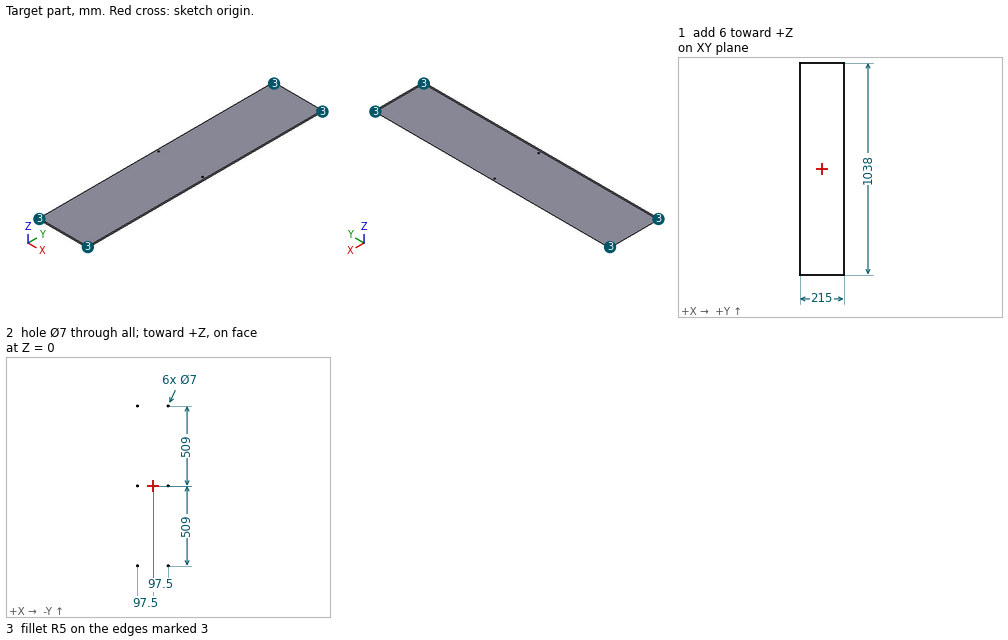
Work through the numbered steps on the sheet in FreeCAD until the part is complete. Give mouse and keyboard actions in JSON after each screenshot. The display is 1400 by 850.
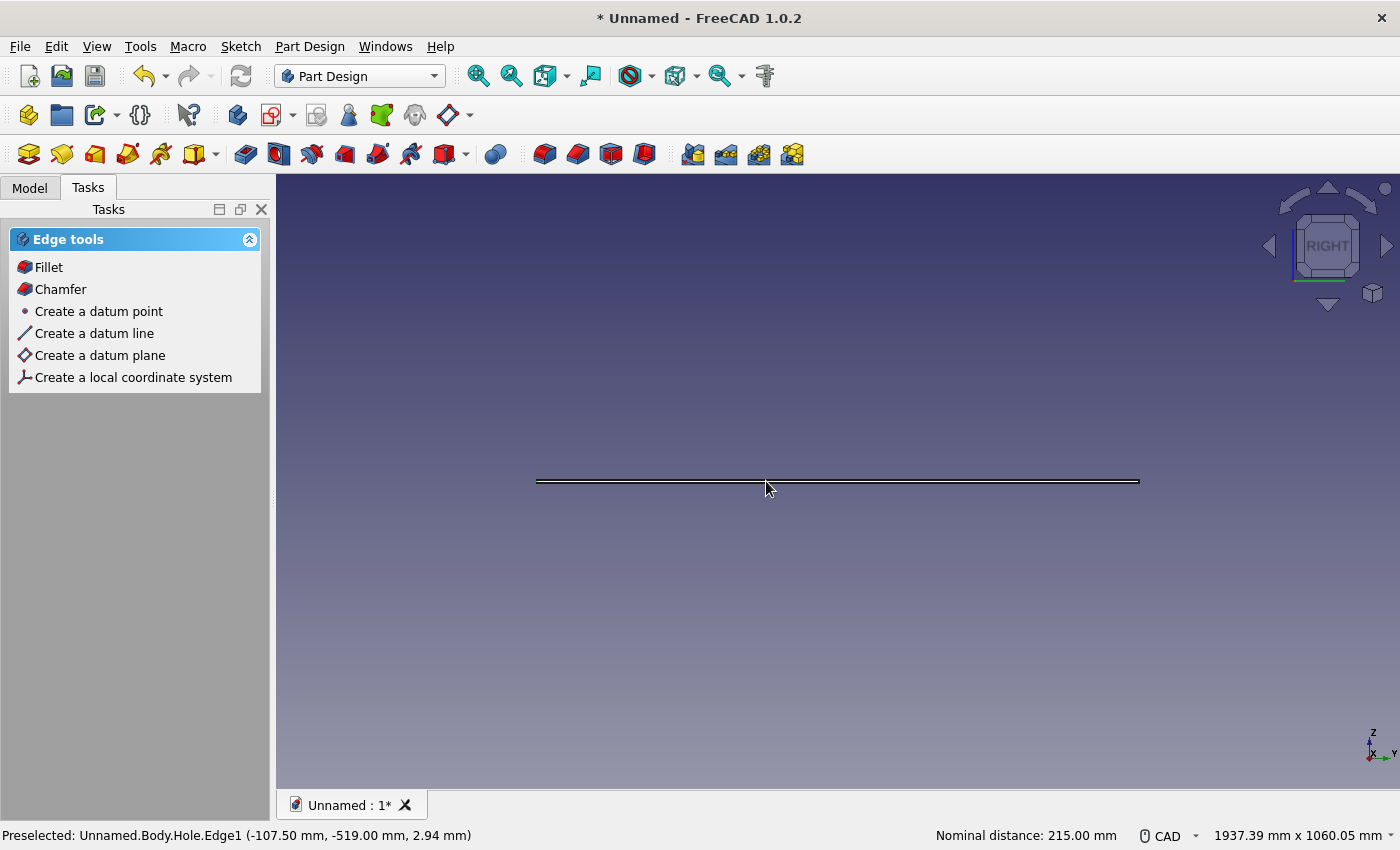
{"action": "scroll", "coordinate": [1139, 480], "scroll_direction": "up", "scroll_amount": 13}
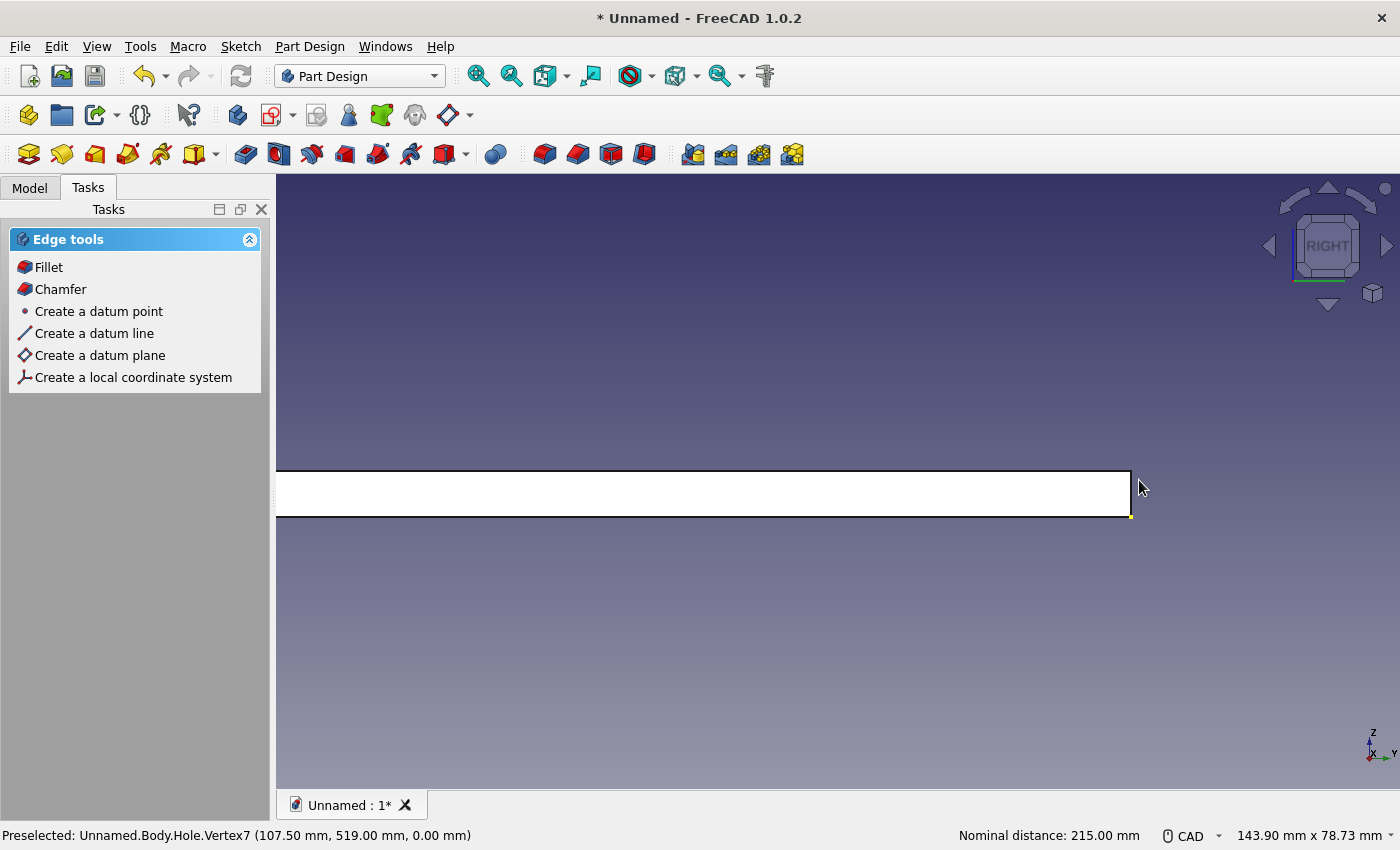
{"action": "left_click", "coordinate": [1131, 493], "text": "ctrl"}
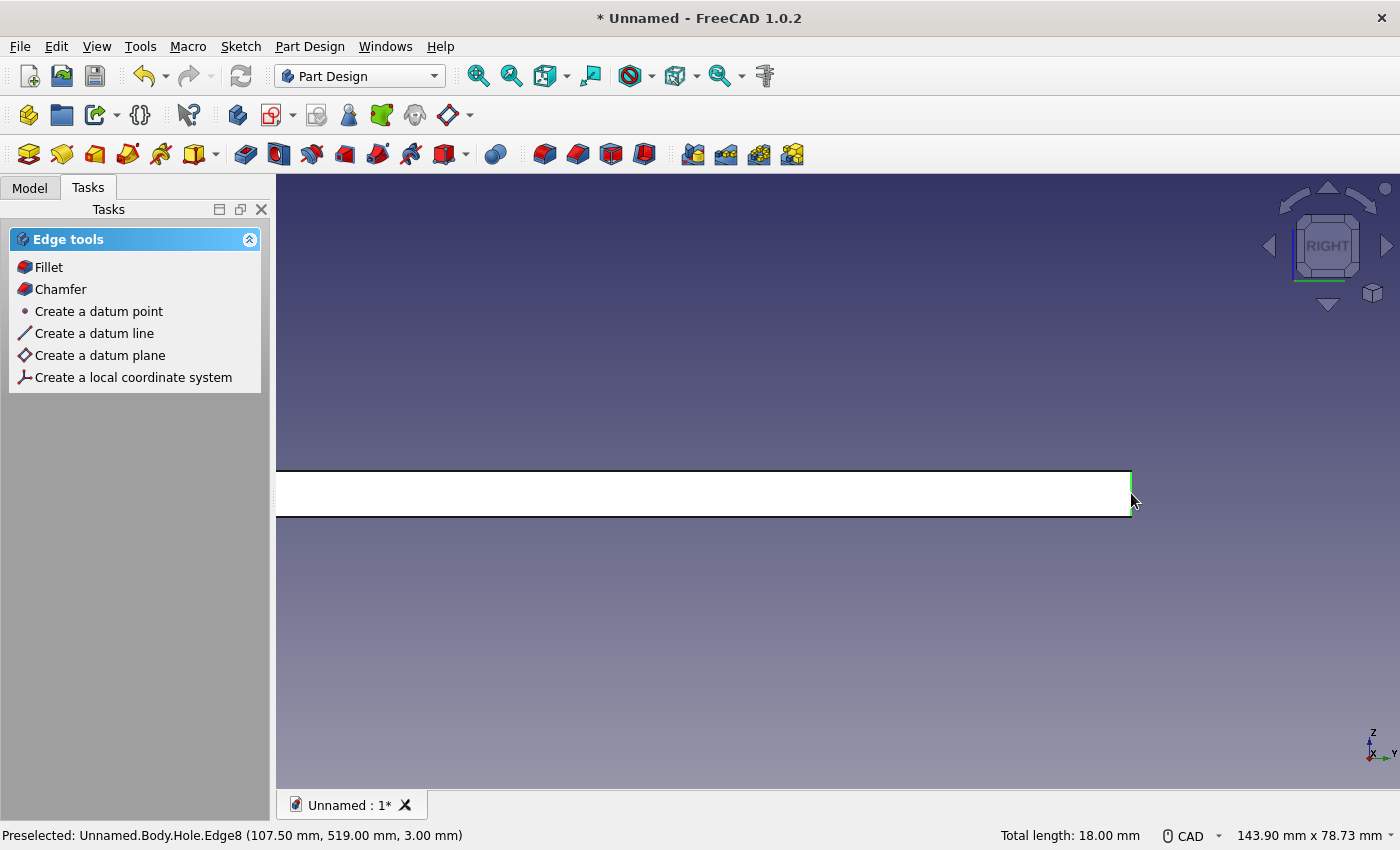
{"action": "left_click", "coordinate": [479, 76]}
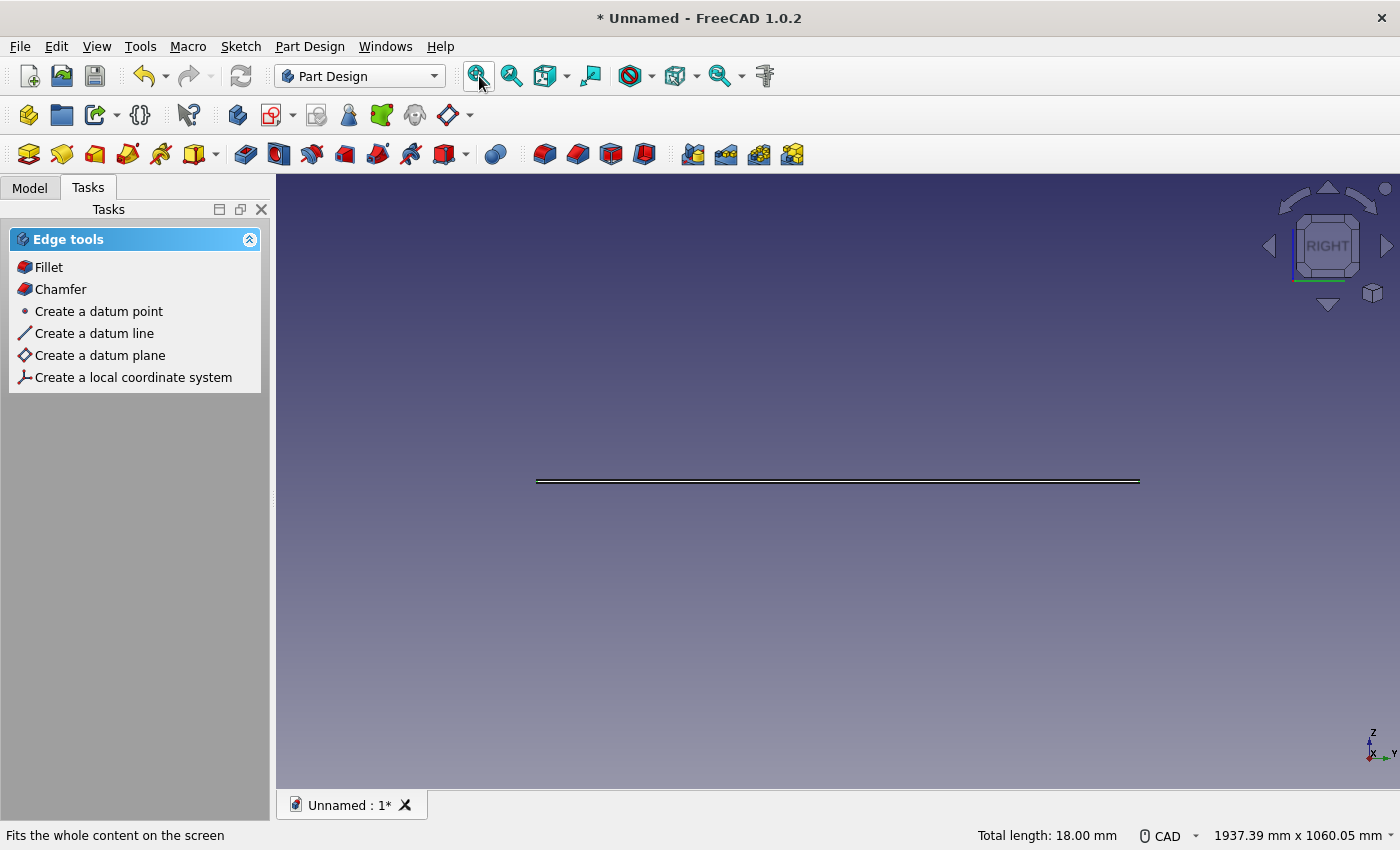
{"action": "key", "text": "5"}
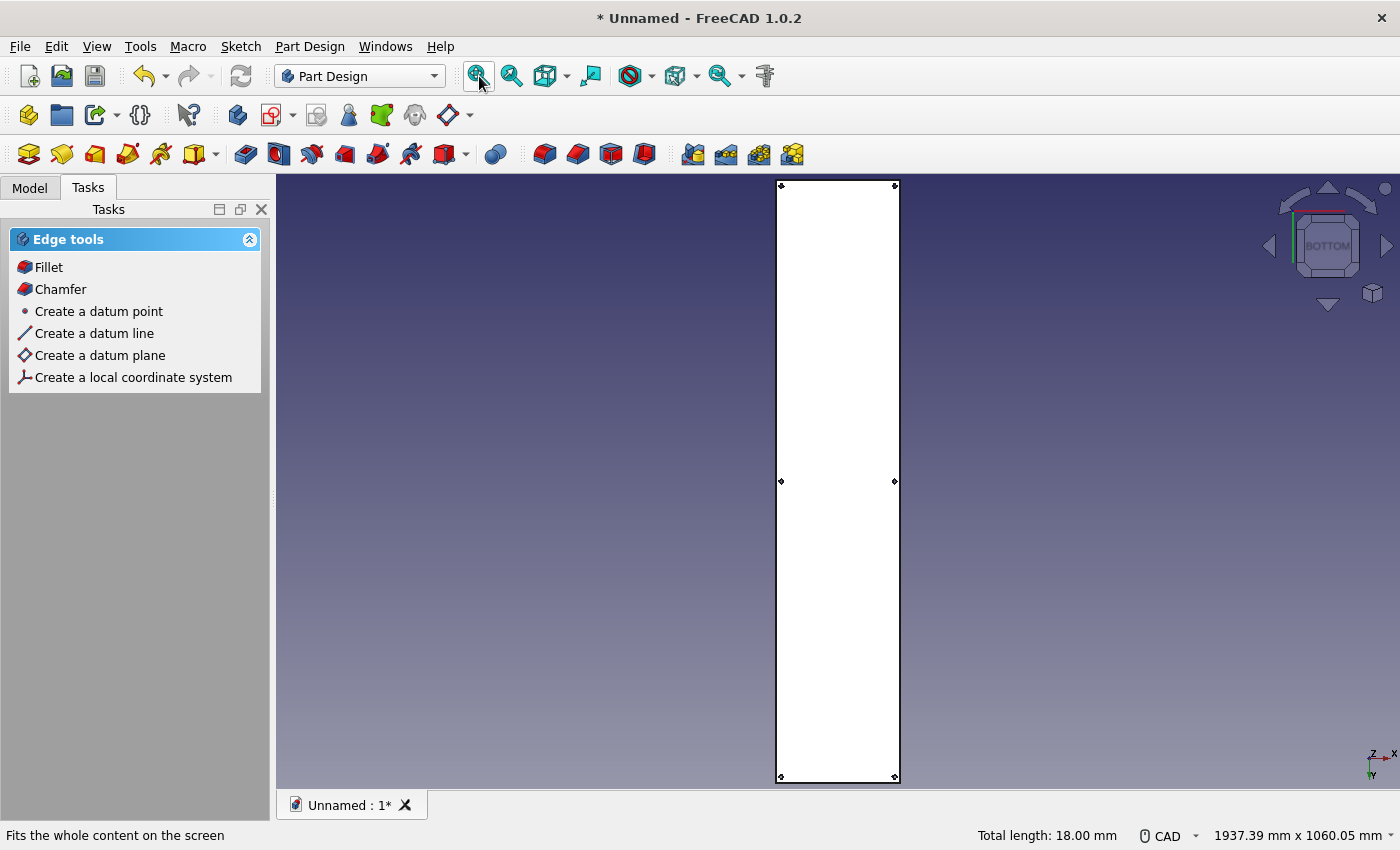
{"action": "key", "text": "4"}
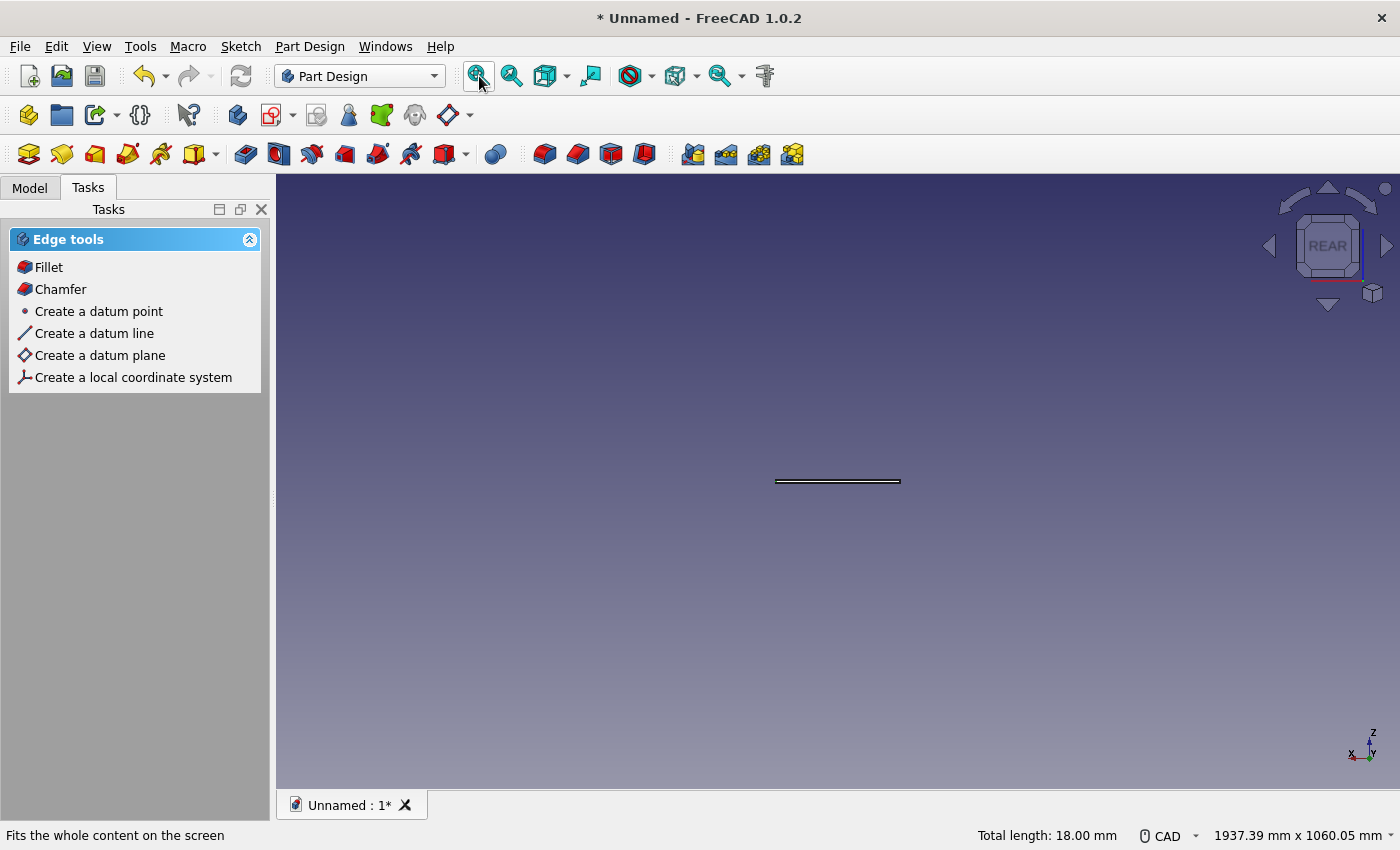
{"action": "key", "text": "v f"}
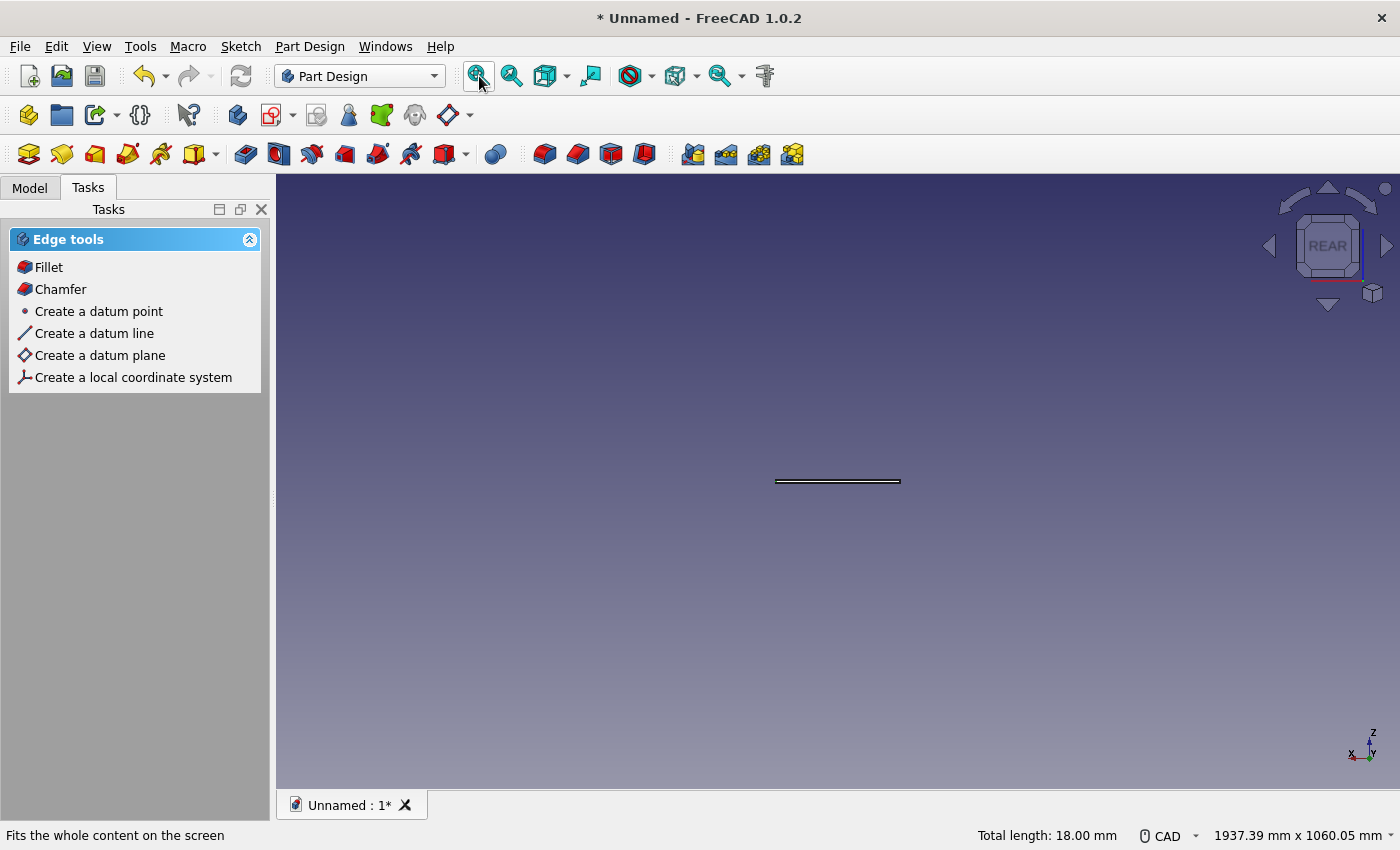
{"action": "scroll", "coordinate": [900, 481], "scroll_direction": "up", "scroll_amount": 13}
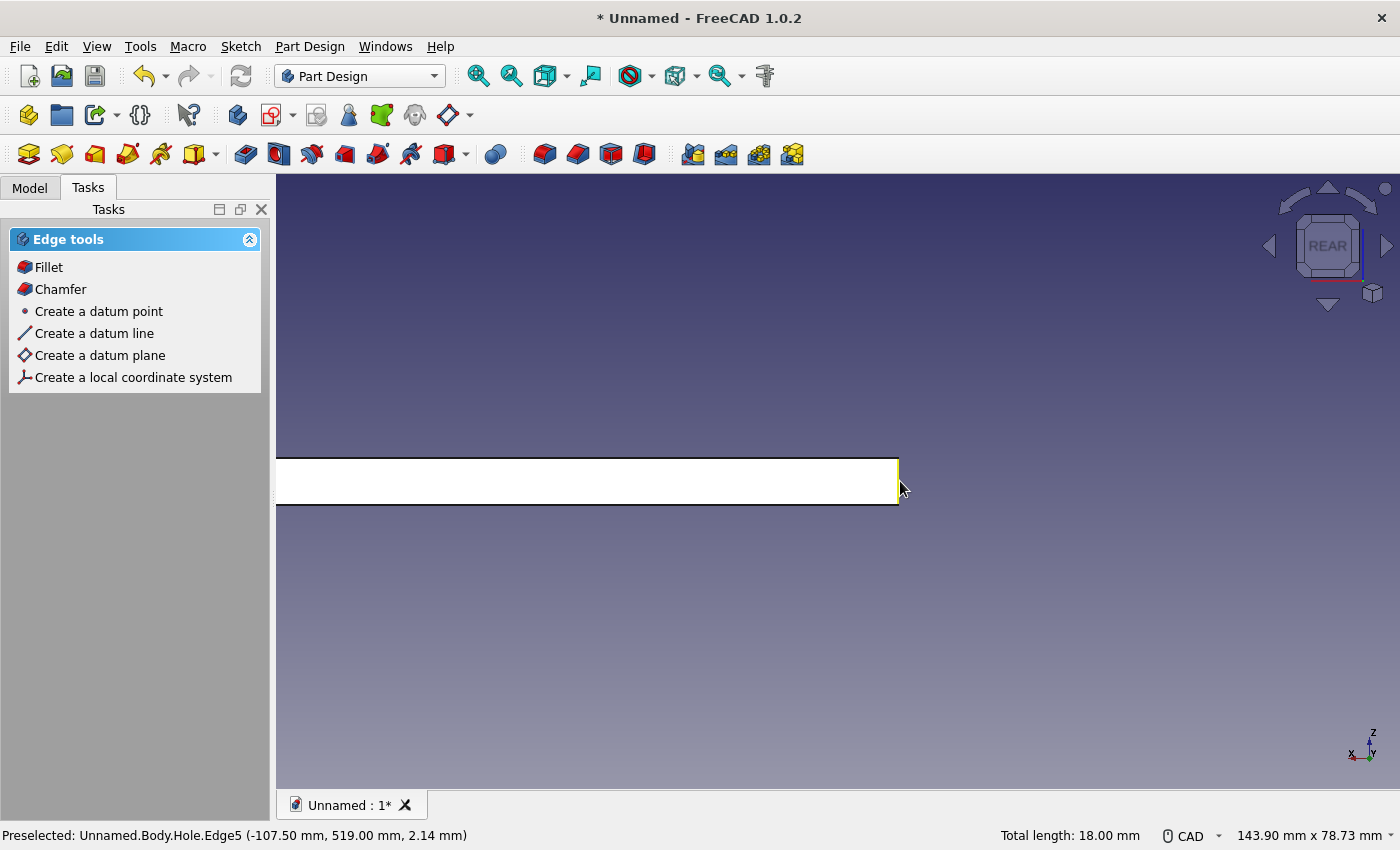
{"action": "left_click", "coordinate": [898, 481], "text": "ctrl"}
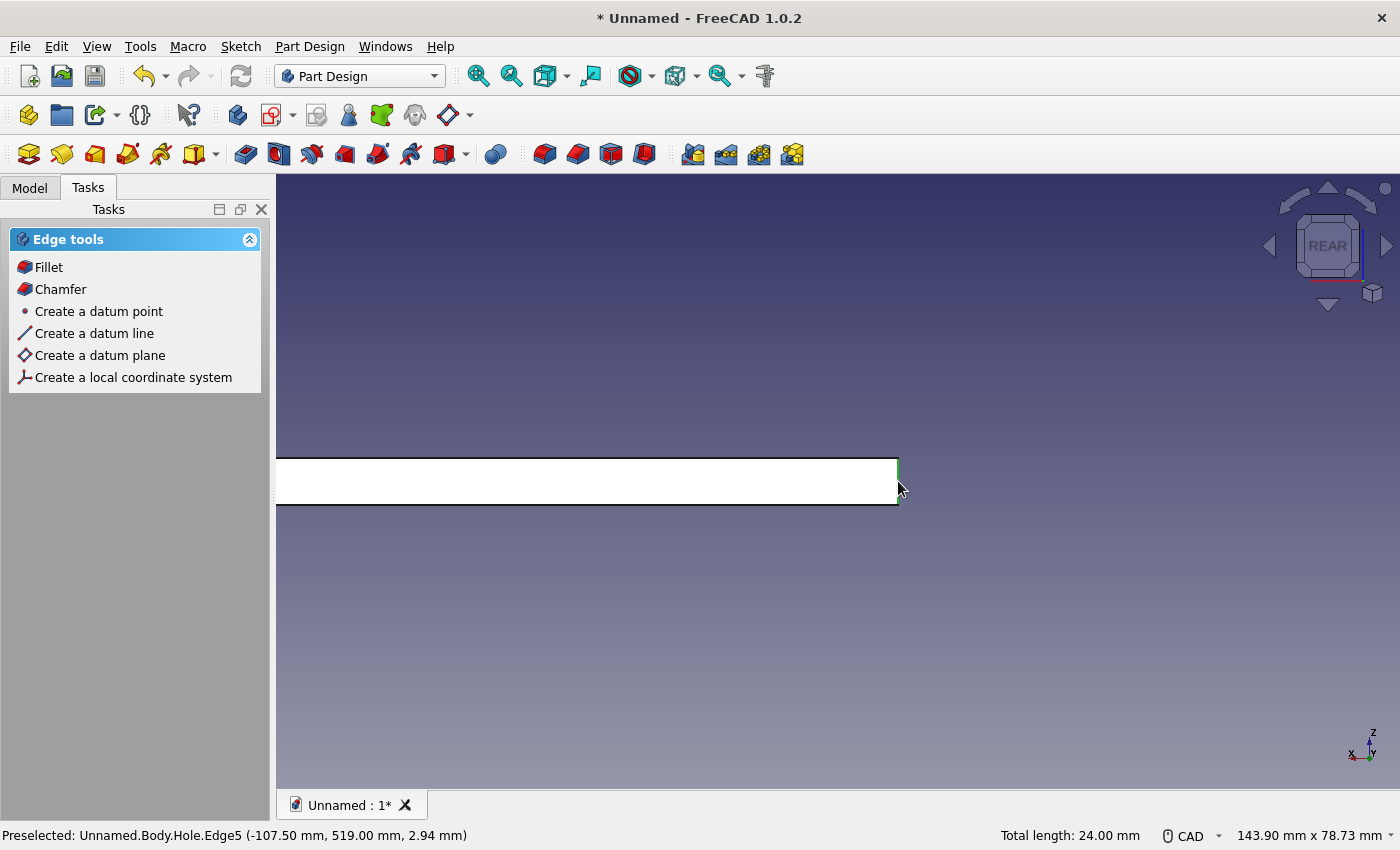
{"action": "left_click", "coordinate": [545, 154]}